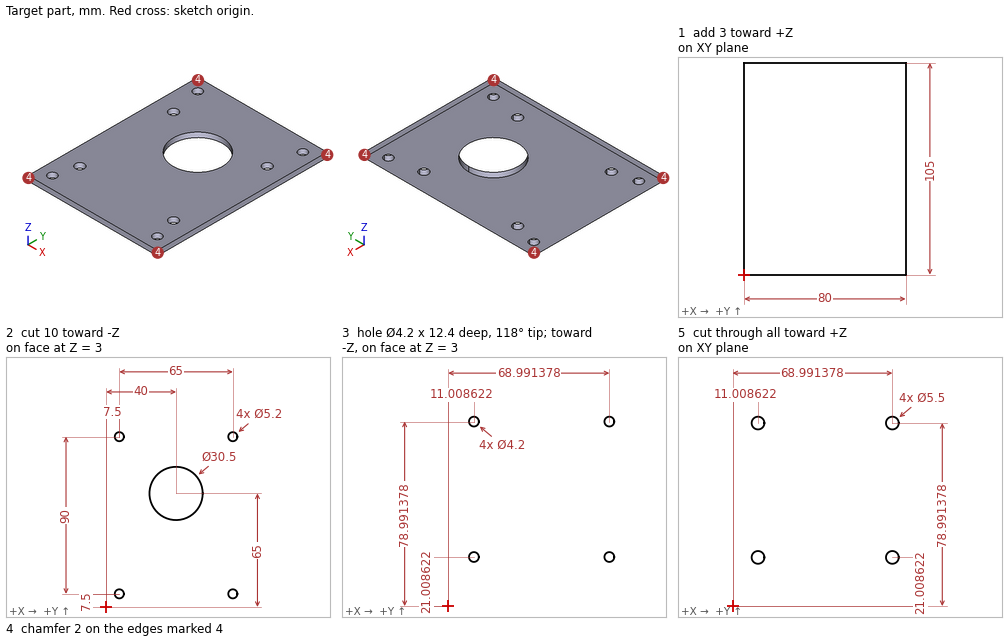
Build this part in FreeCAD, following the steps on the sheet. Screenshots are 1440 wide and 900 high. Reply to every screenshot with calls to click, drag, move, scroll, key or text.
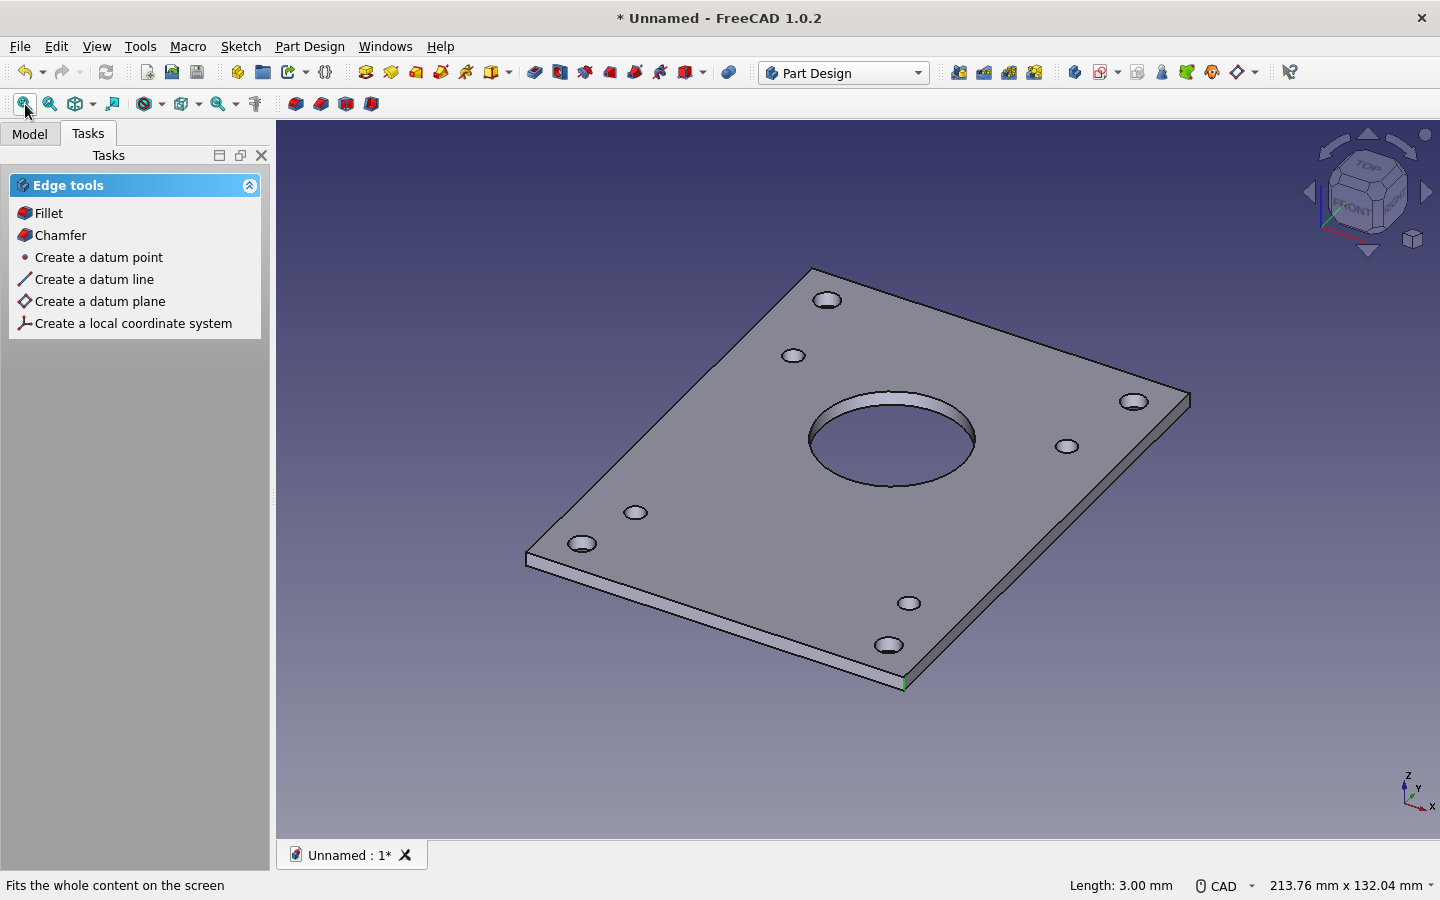
key(0)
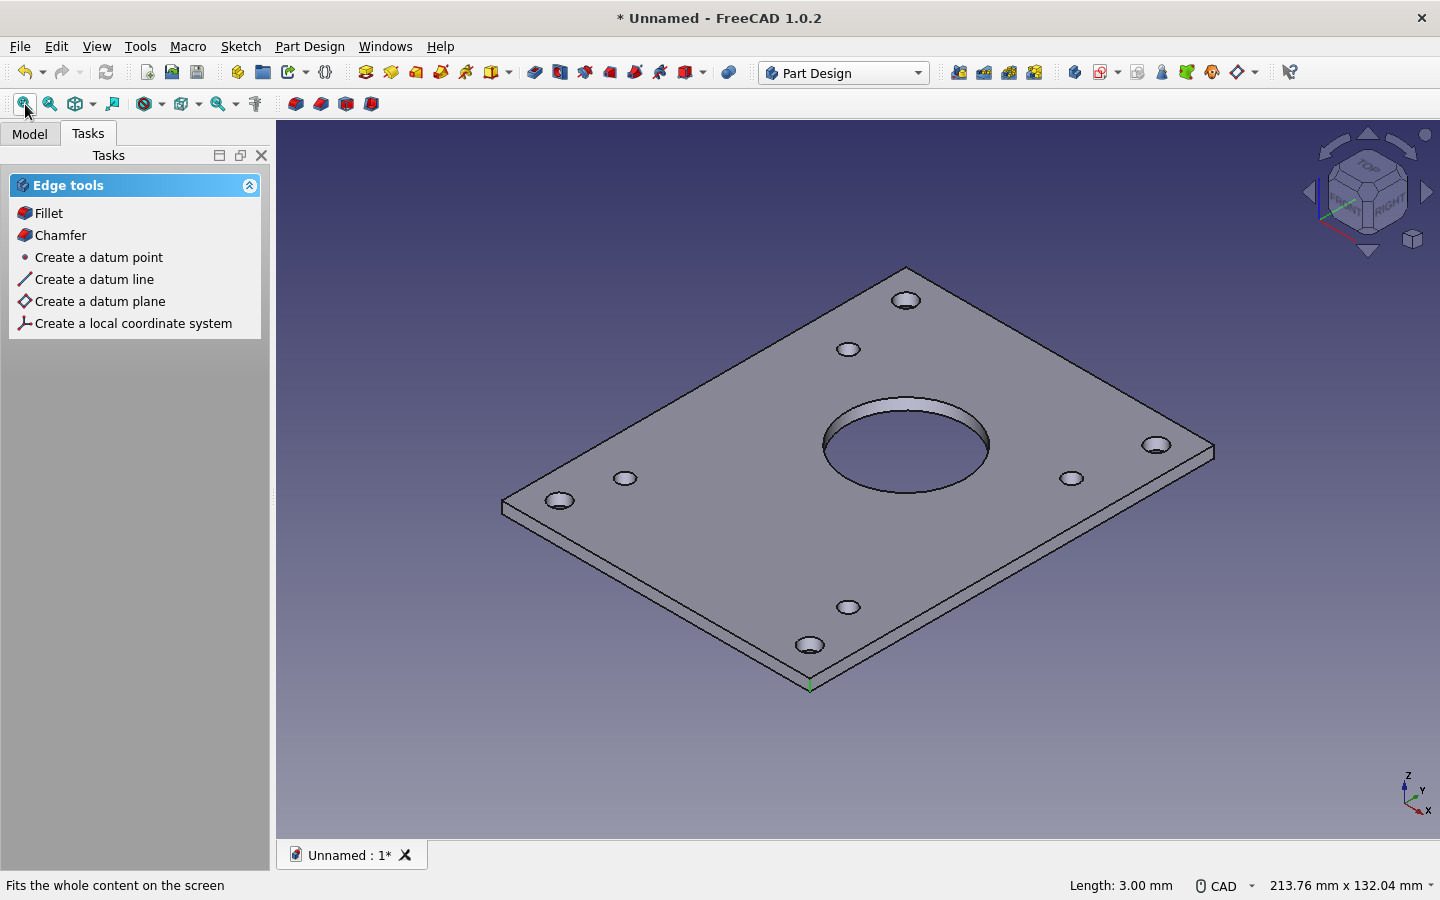
scroll(906, 273, up, 5)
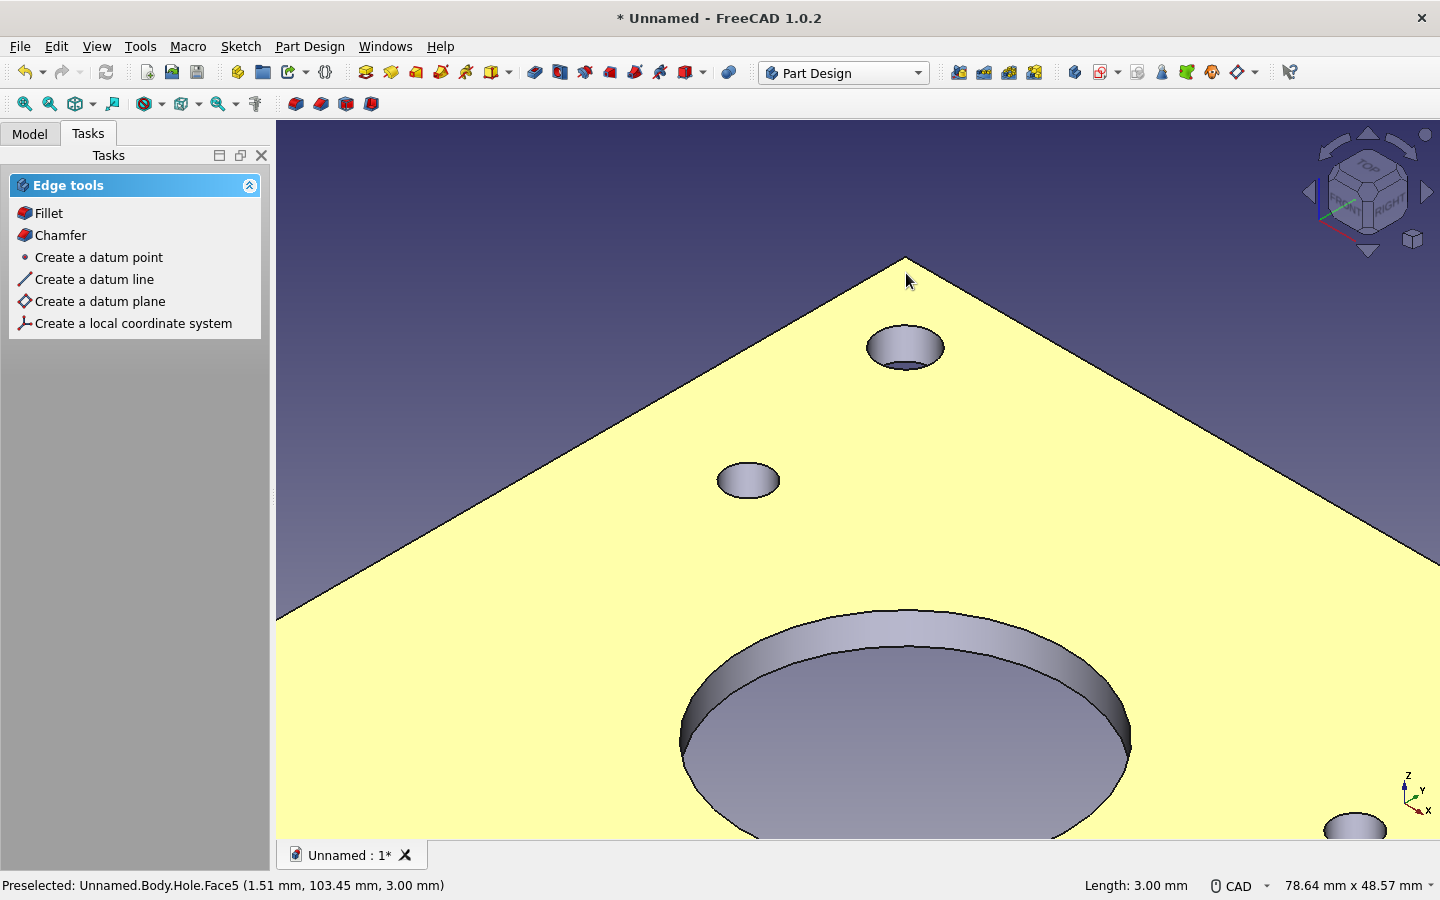
click(25, 104)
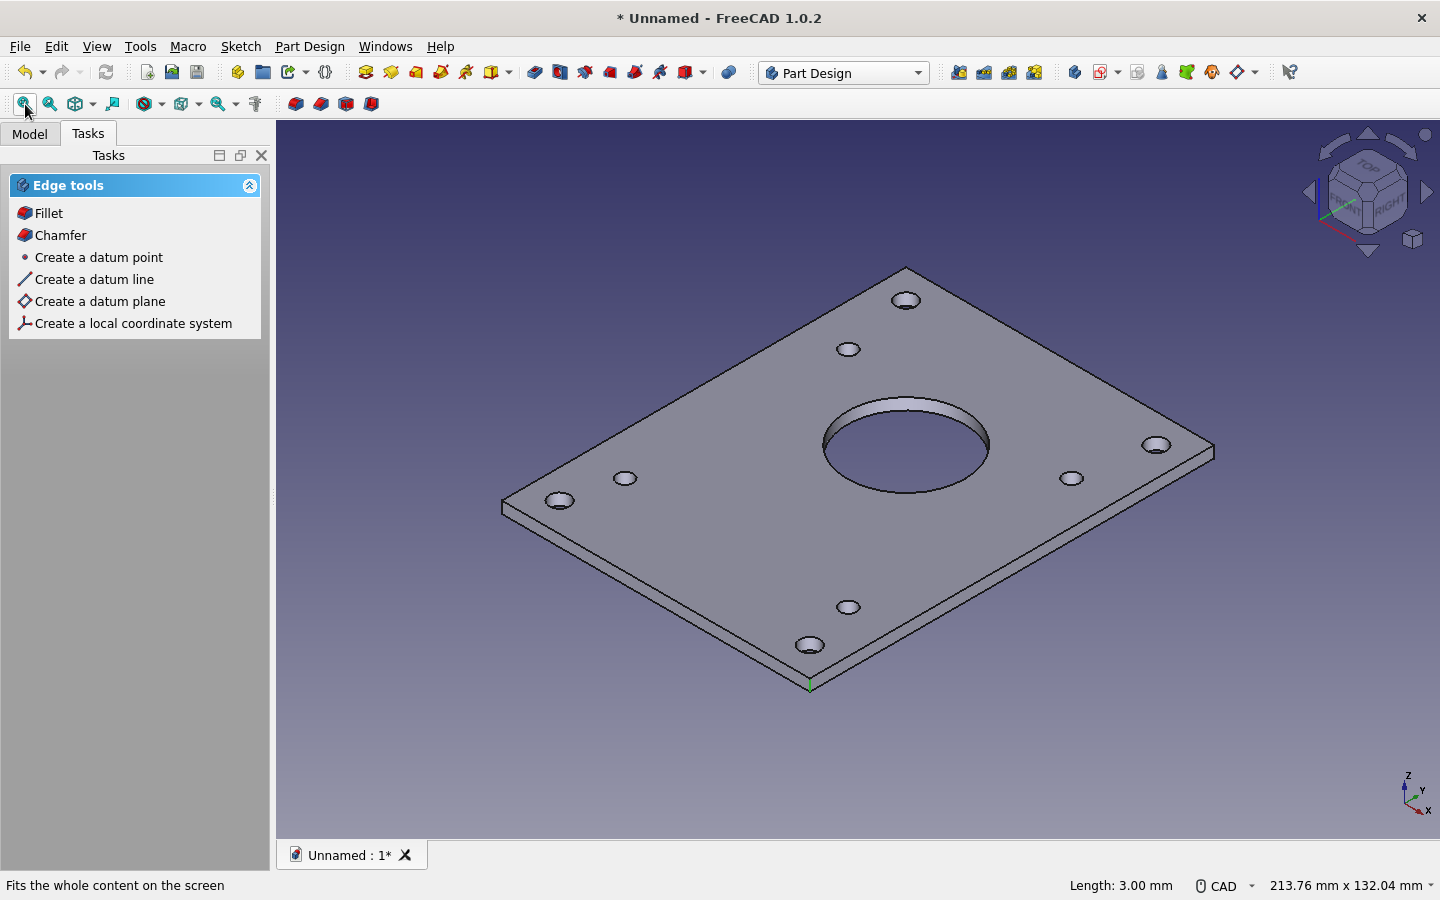
key(2)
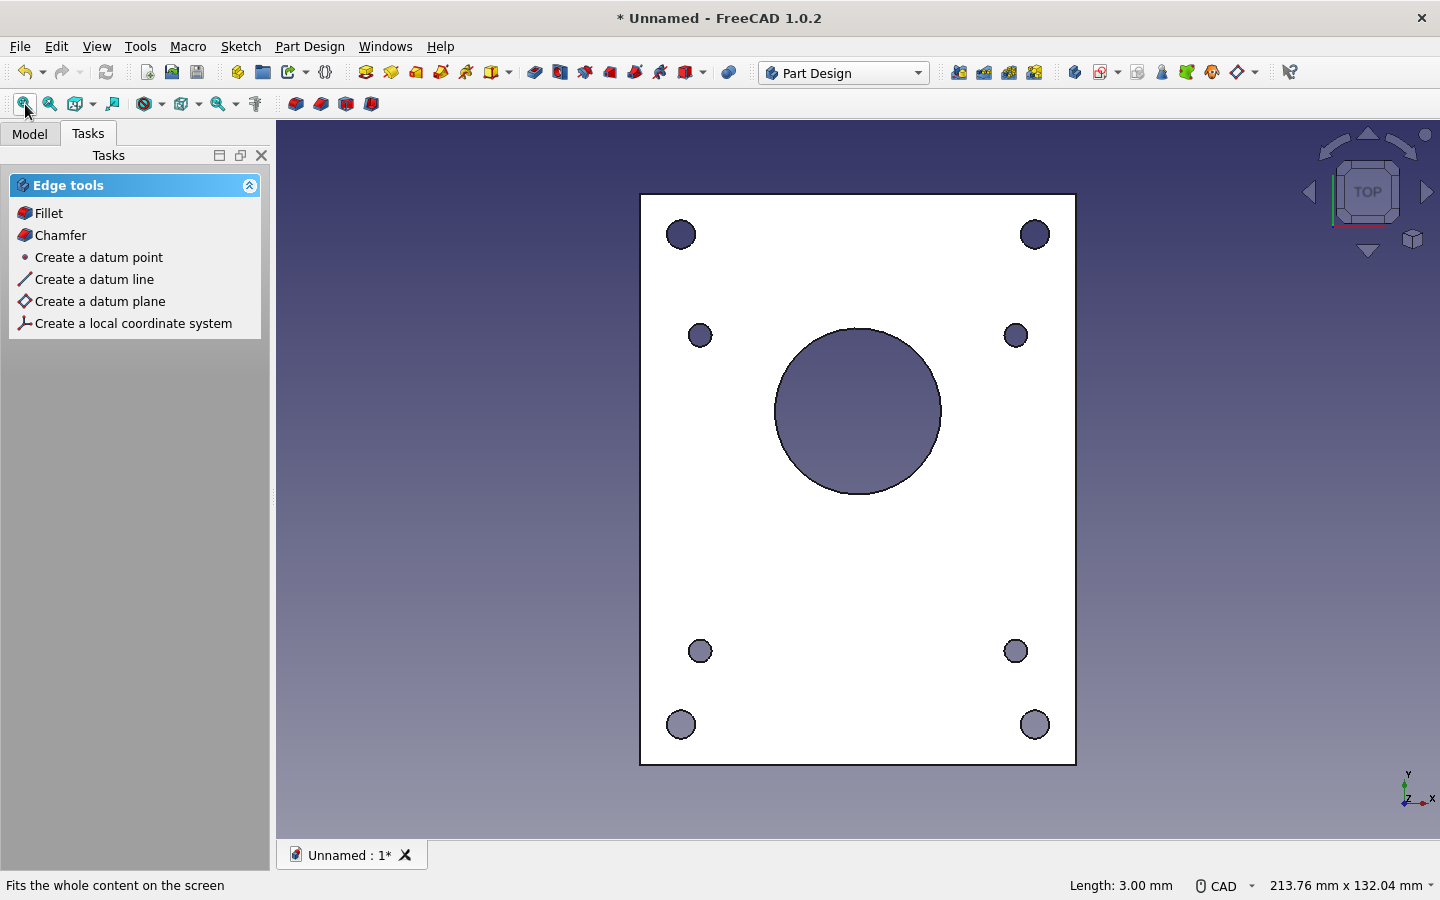
scroll(640, 193, up, 5)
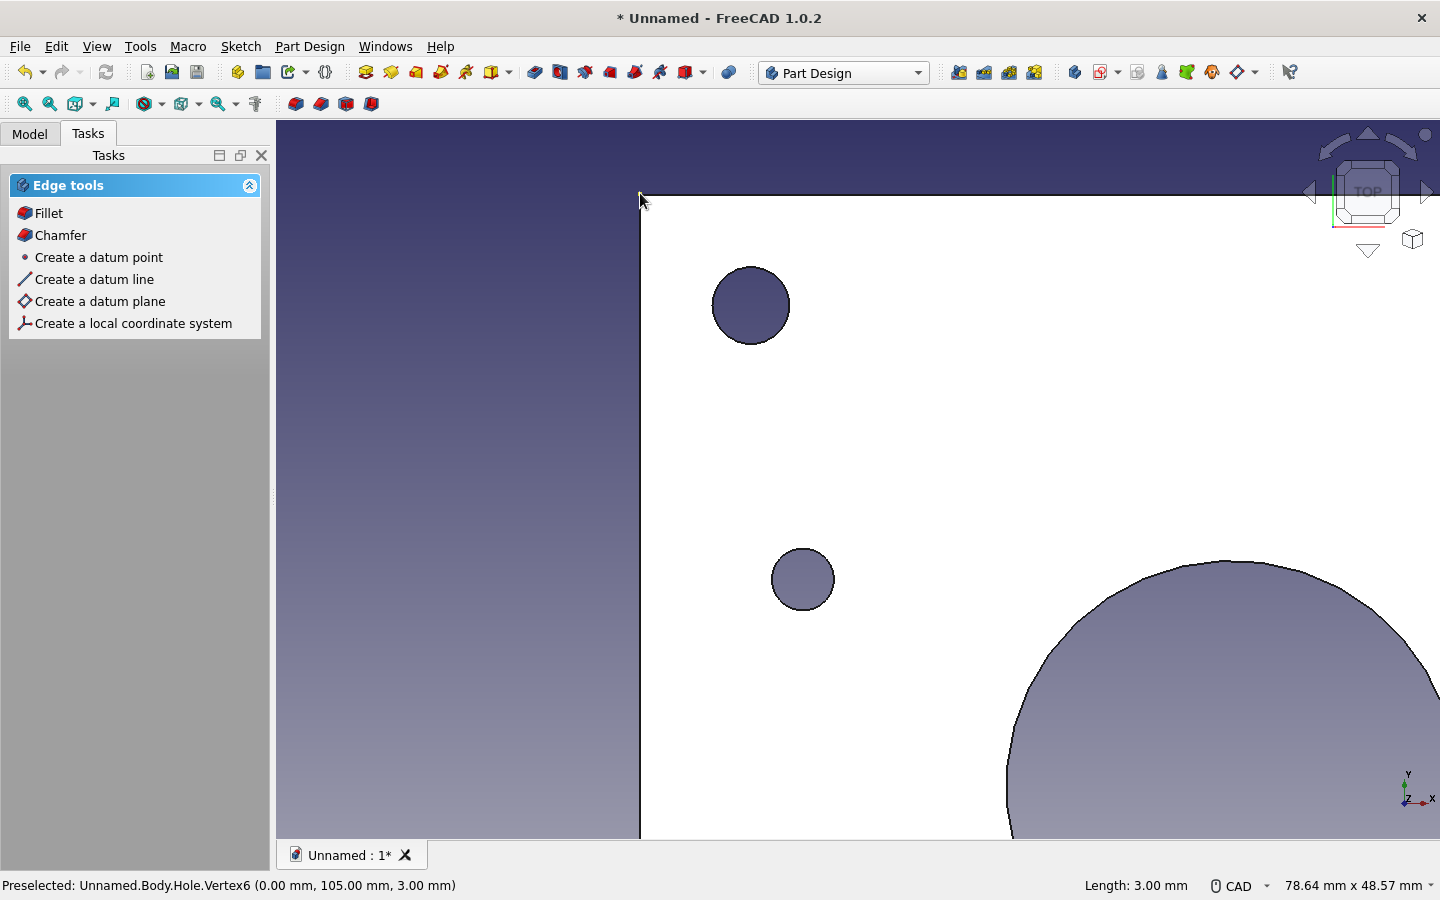
click(25, 104)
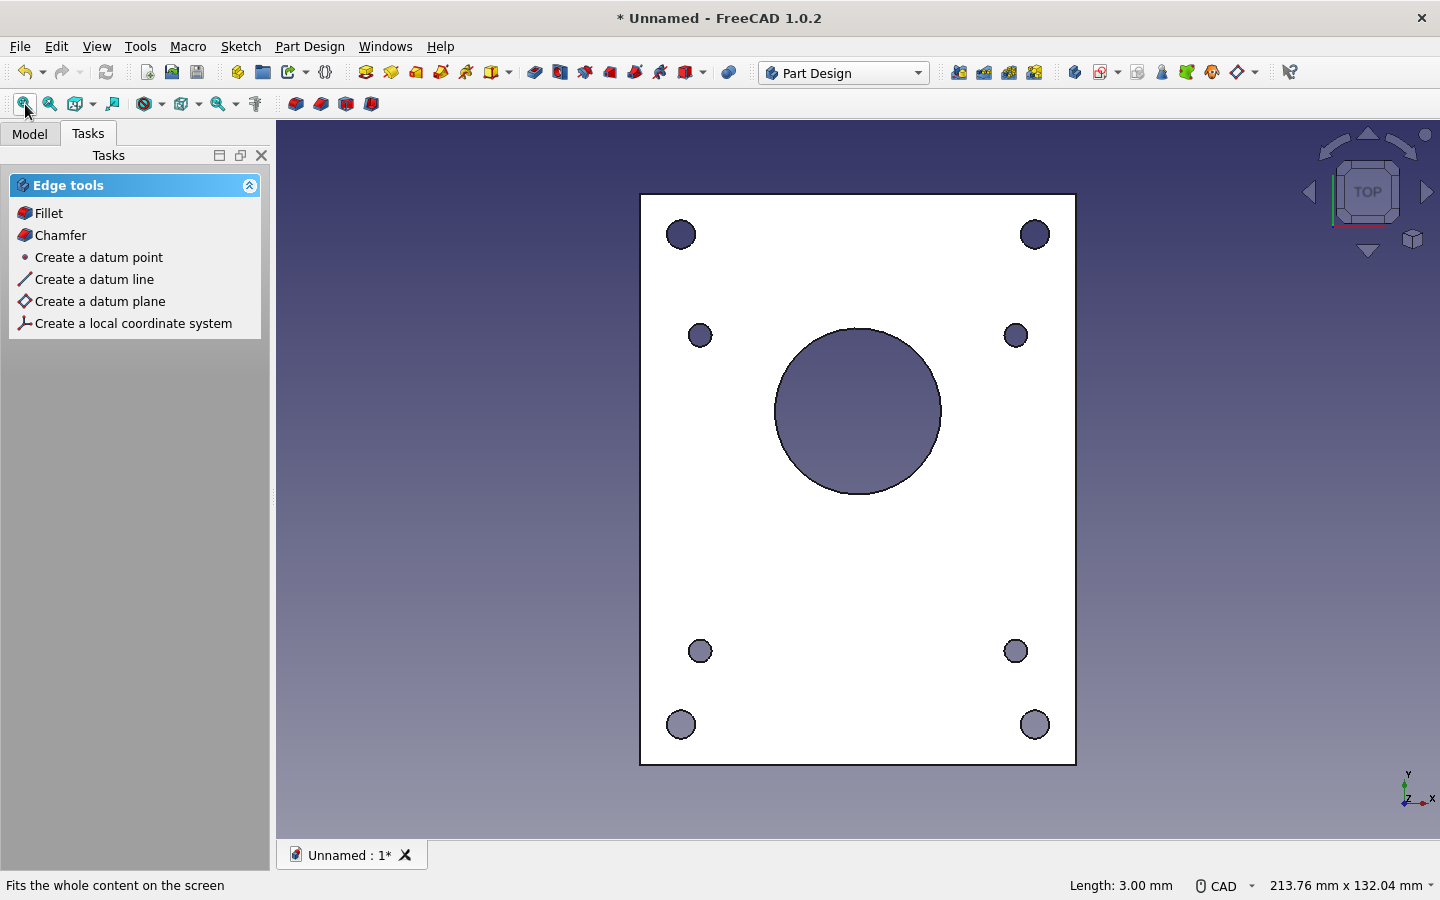
key(1)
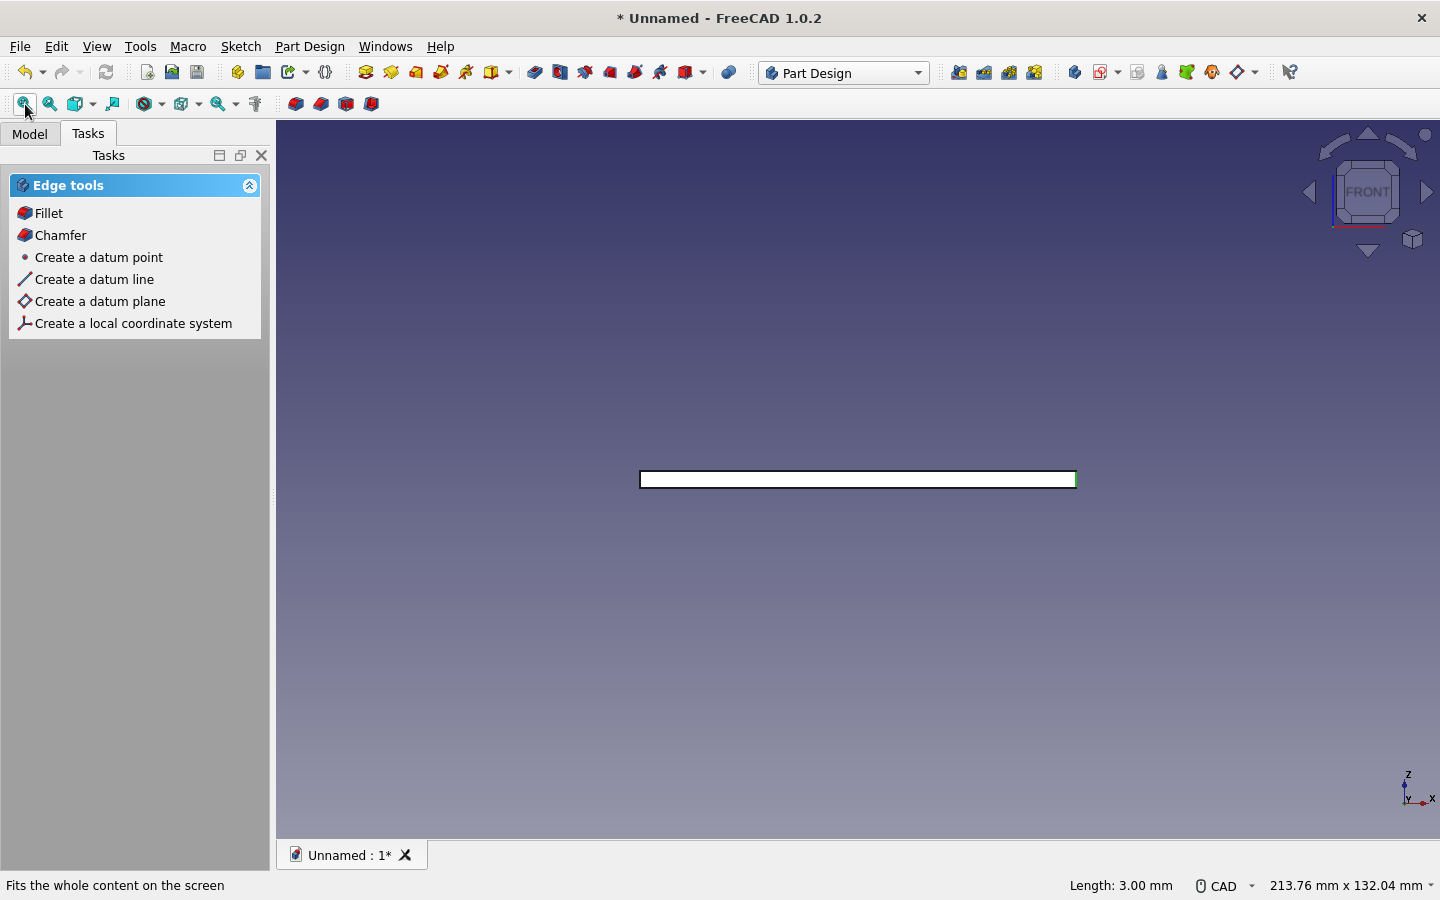
click(25, 104)